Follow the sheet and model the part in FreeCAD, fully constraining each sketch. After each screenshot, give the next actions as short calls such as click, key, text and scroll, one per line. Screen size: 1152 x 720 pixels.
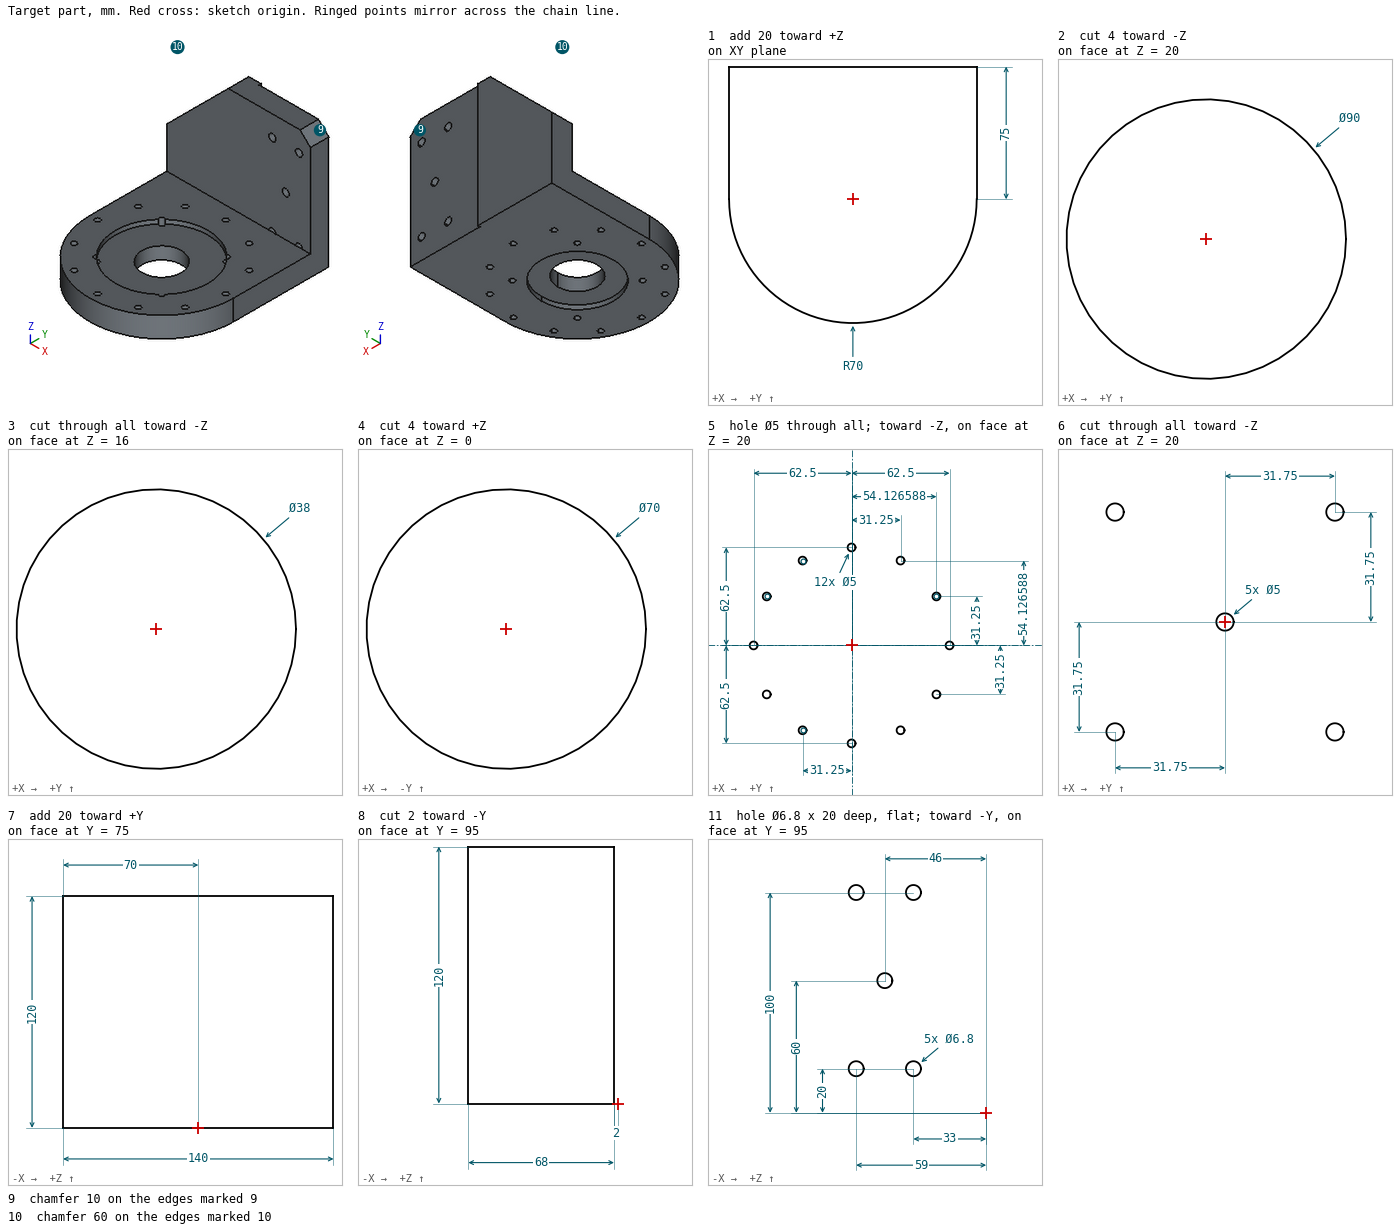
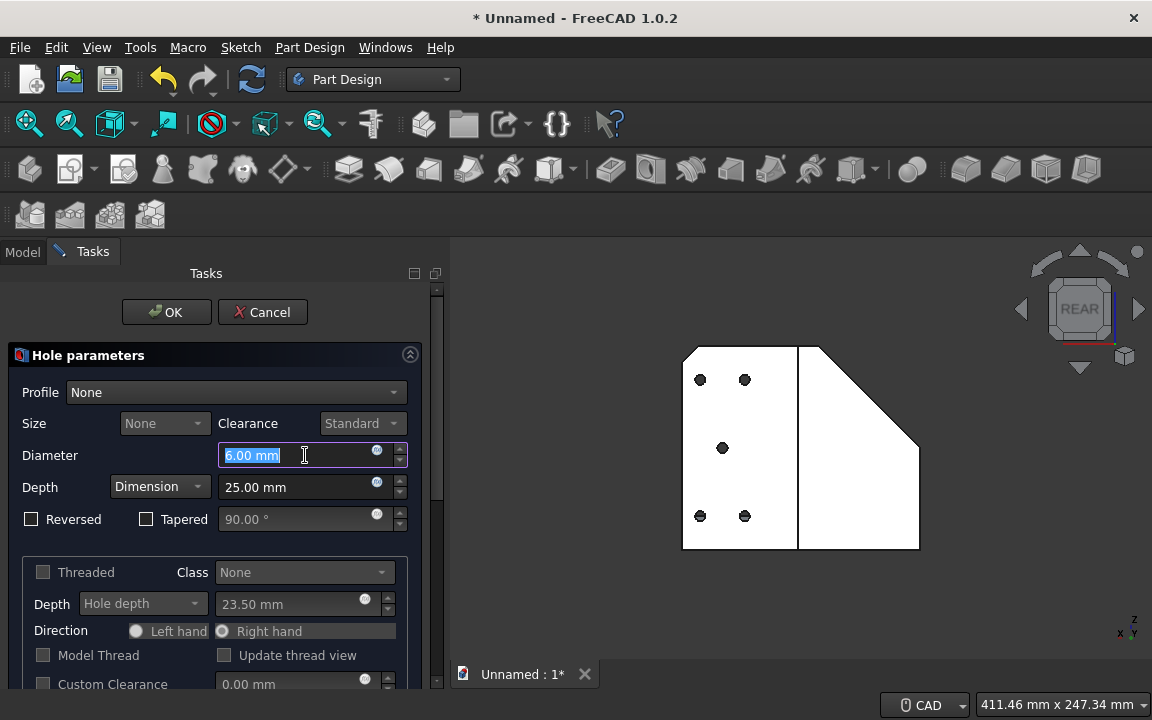
text(6.8)
key(Tab)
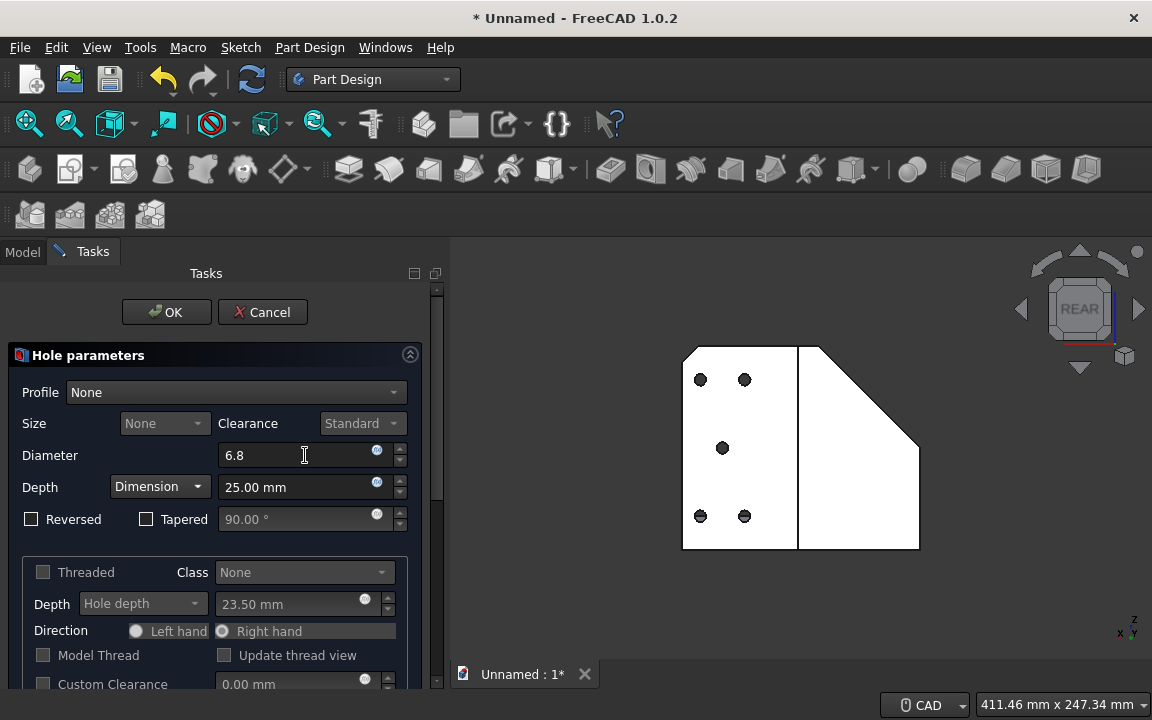
triple_click(305, 487)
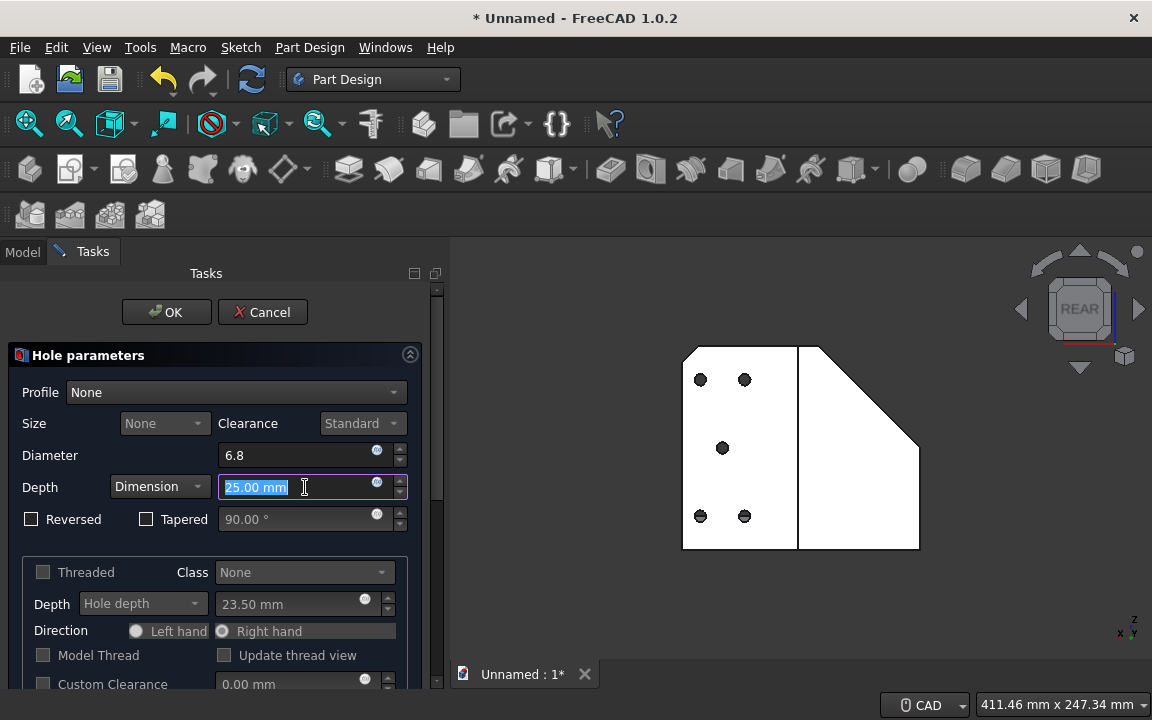
text(20)
key(Tab)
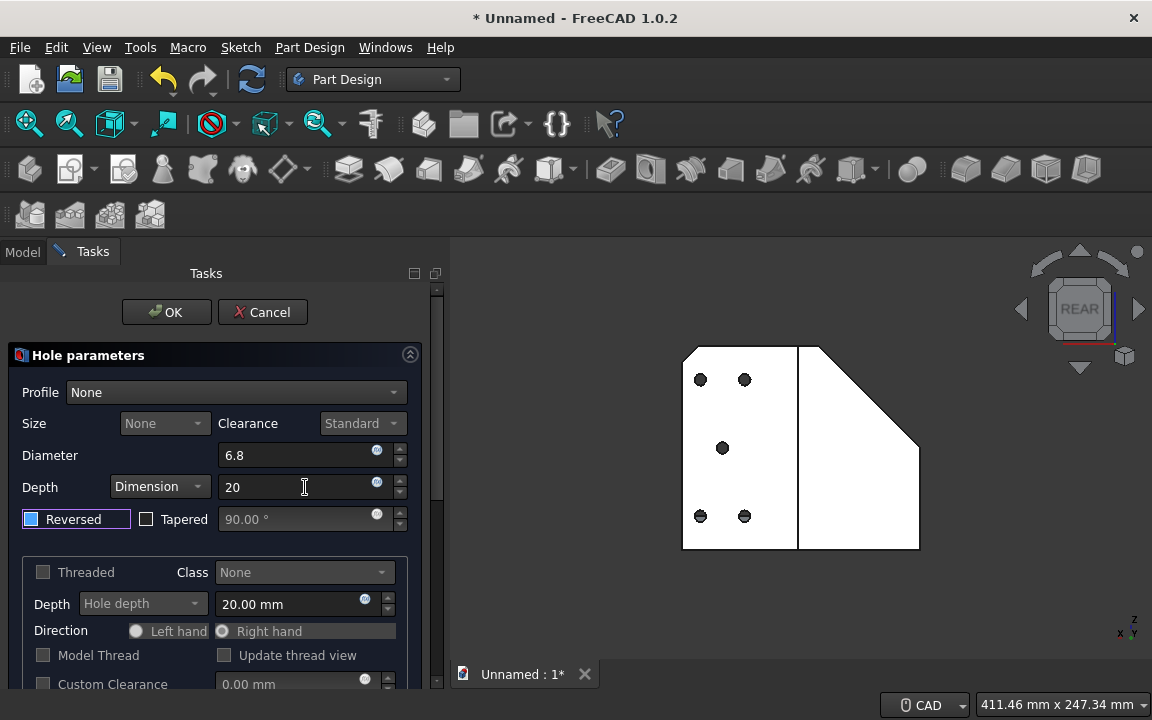
scroll(437, 486, down, 6)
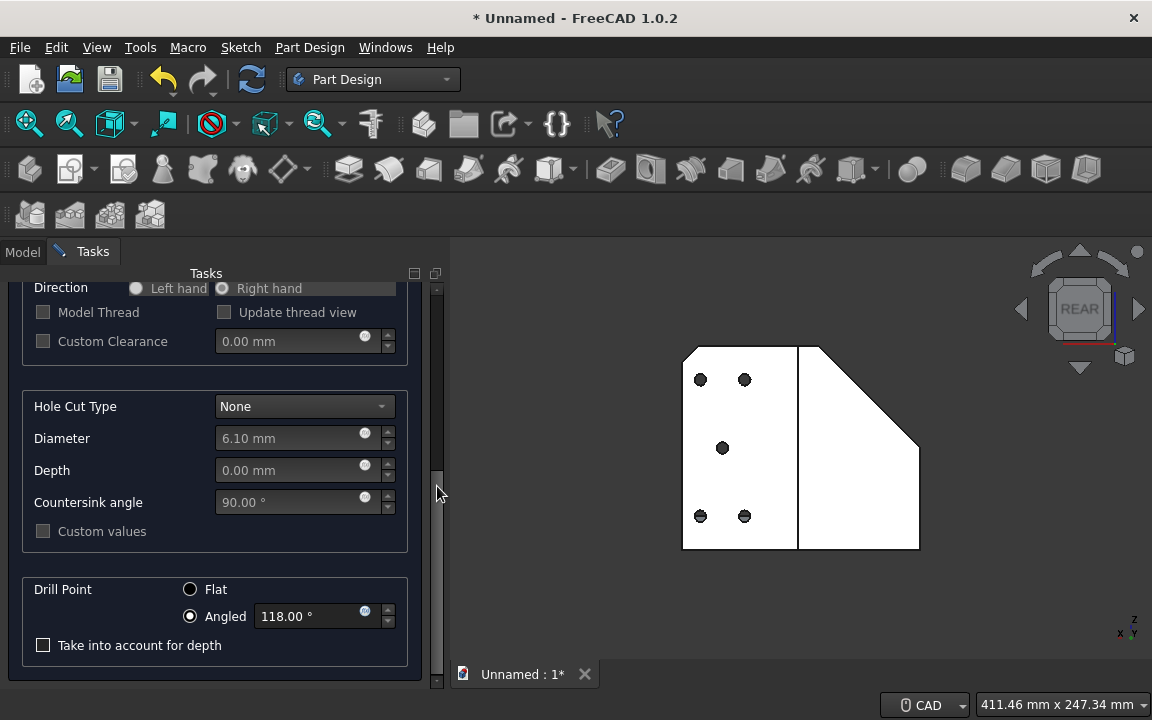
click(191, 589)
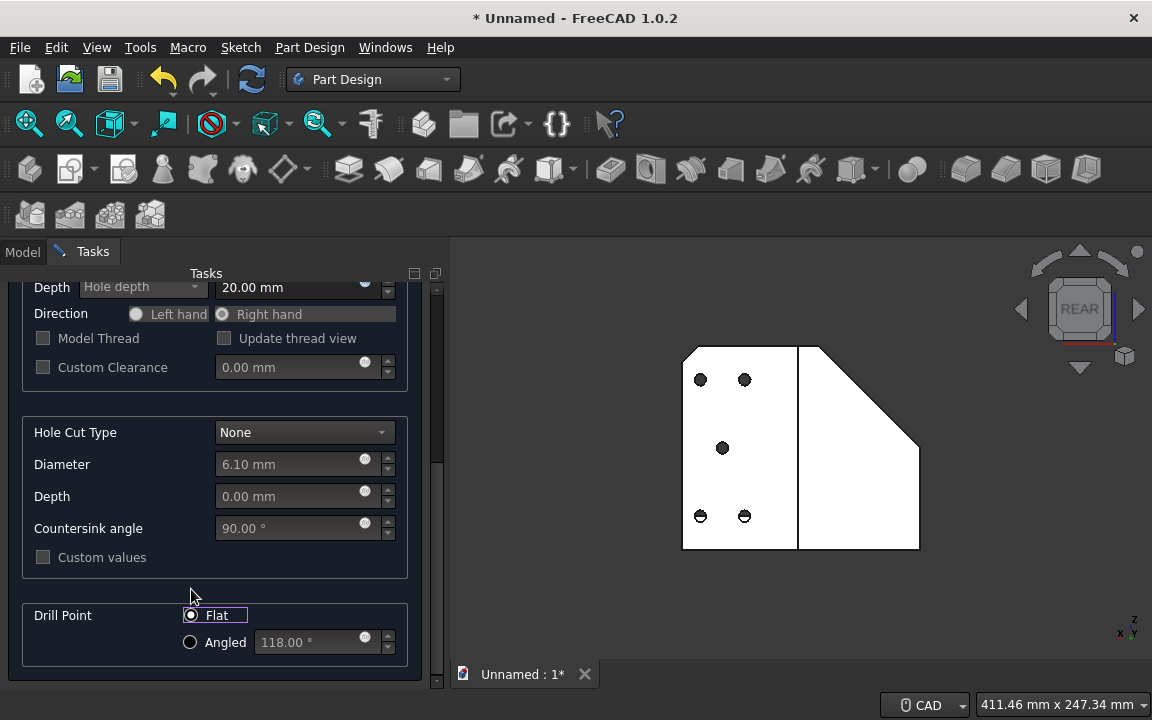
scroll(437, 486, up, 7)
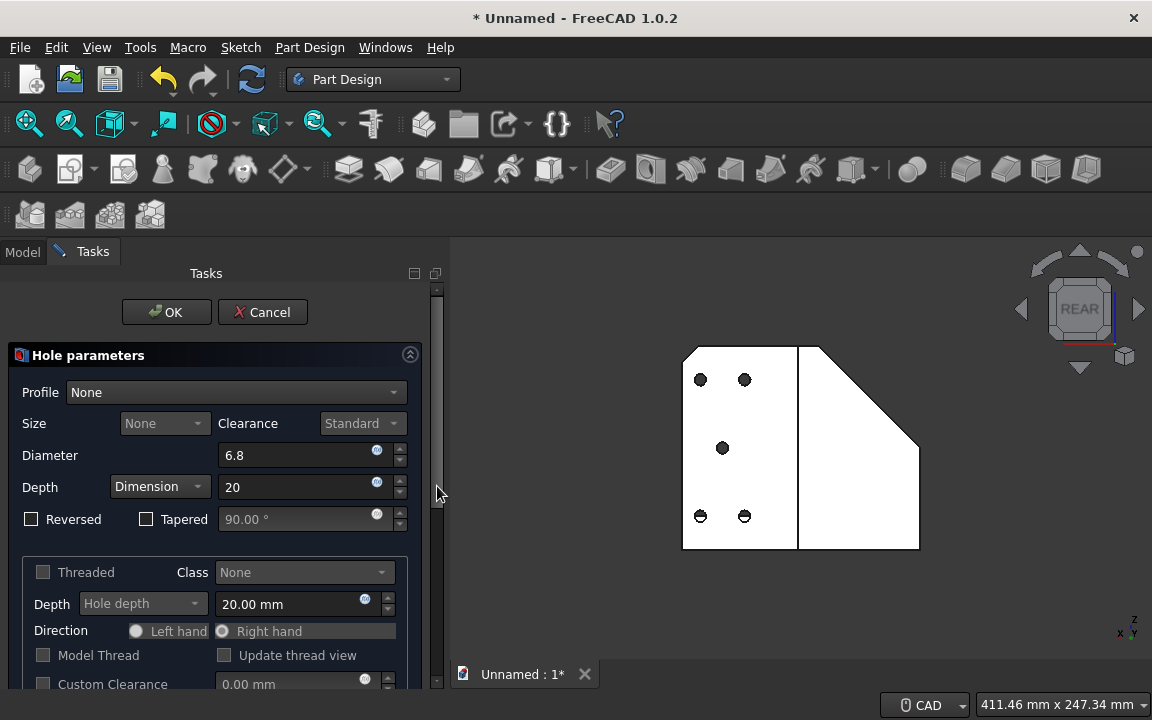
click(167, 312)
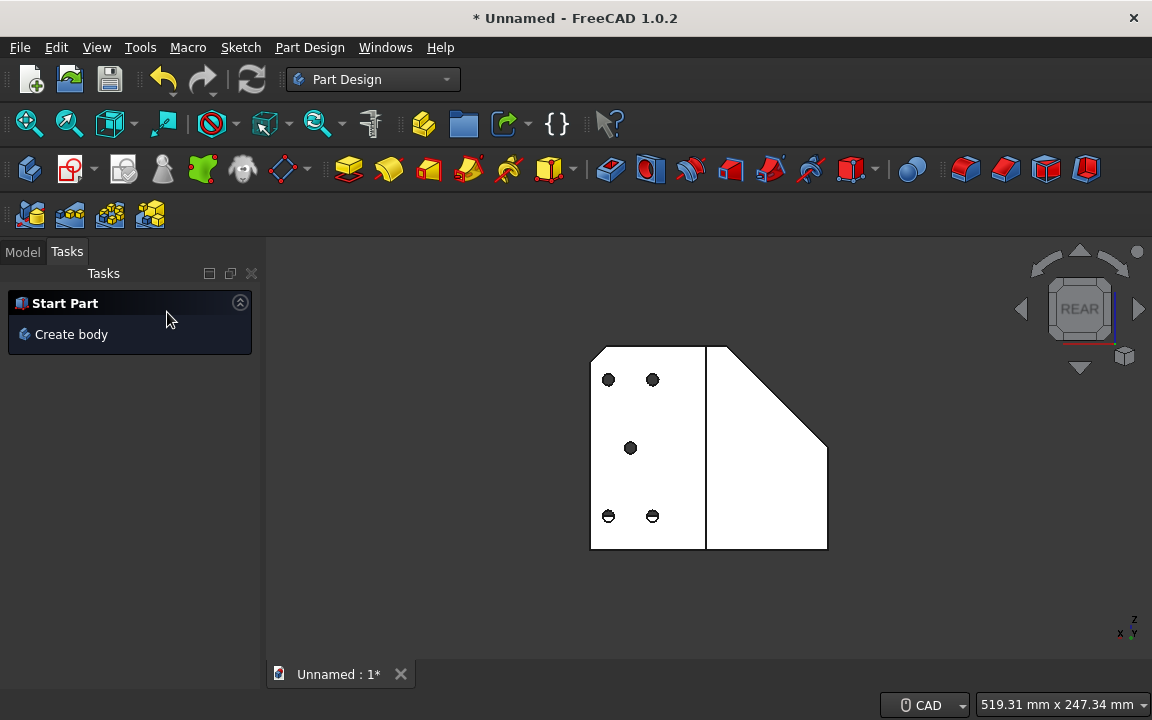
key(0)